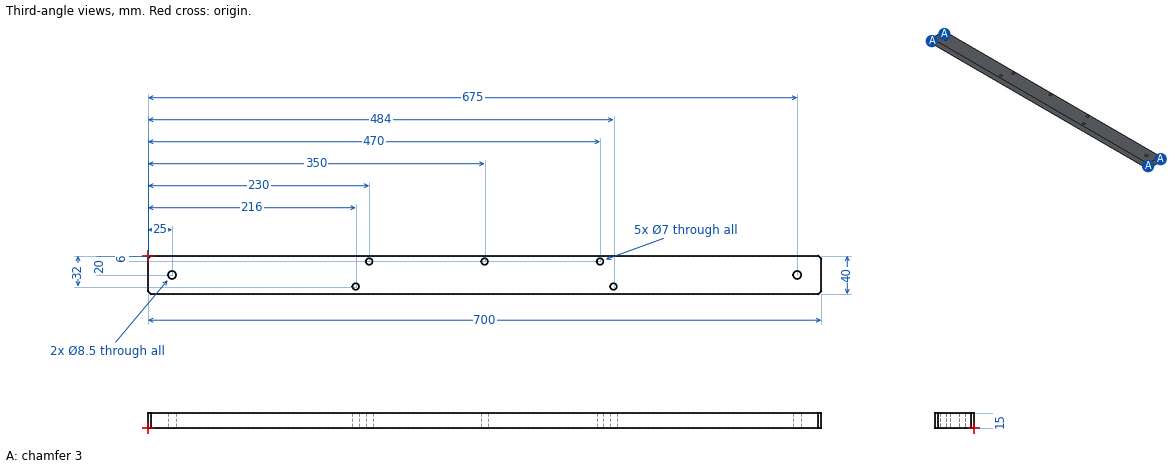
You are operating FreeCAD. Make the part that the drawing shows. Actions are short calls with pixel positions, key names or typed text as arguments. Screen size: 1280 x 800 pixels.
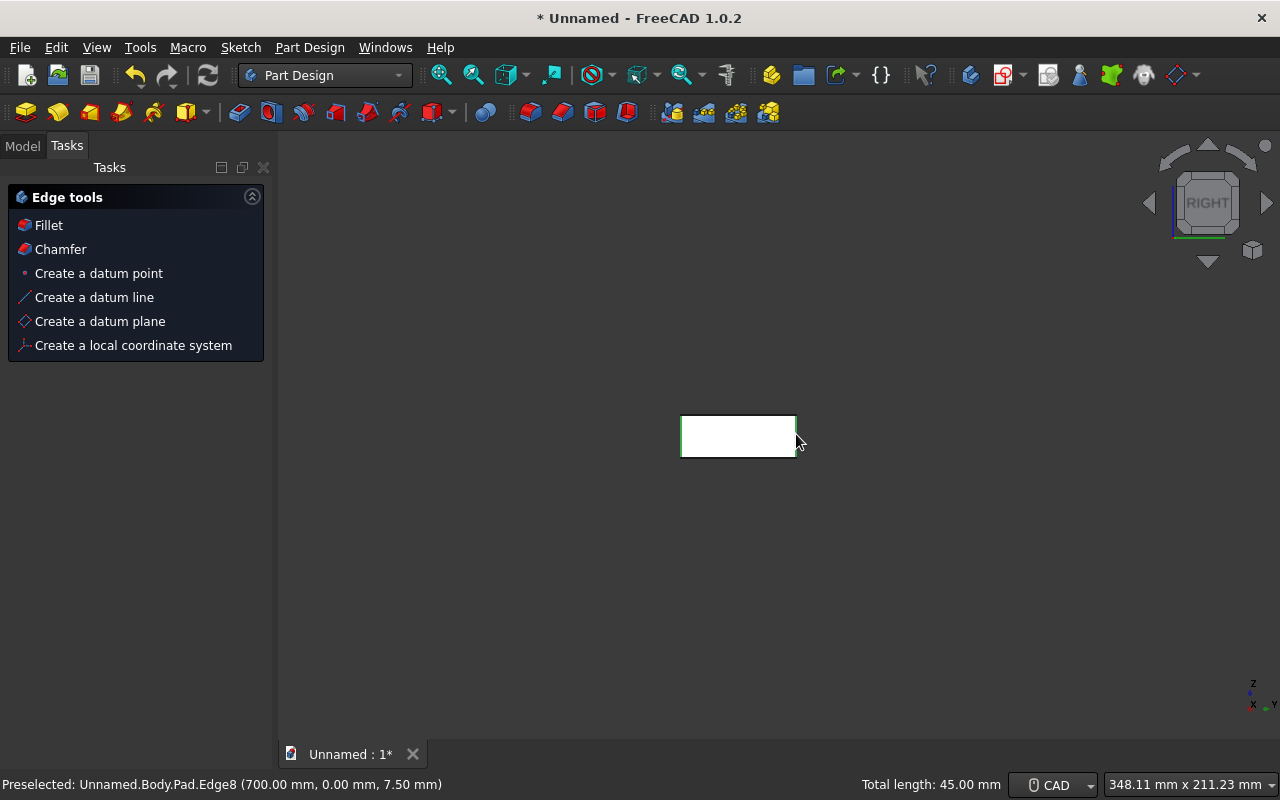
click(442, 76)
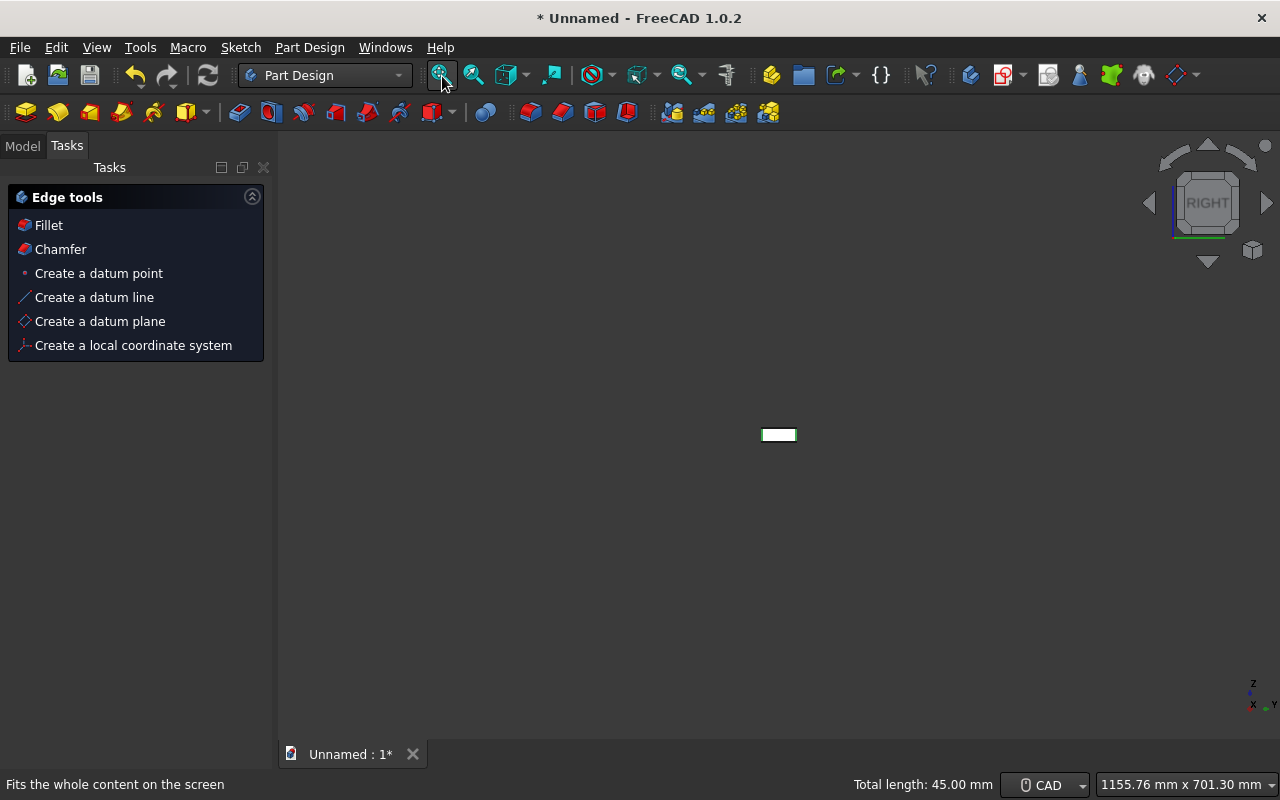
key(5)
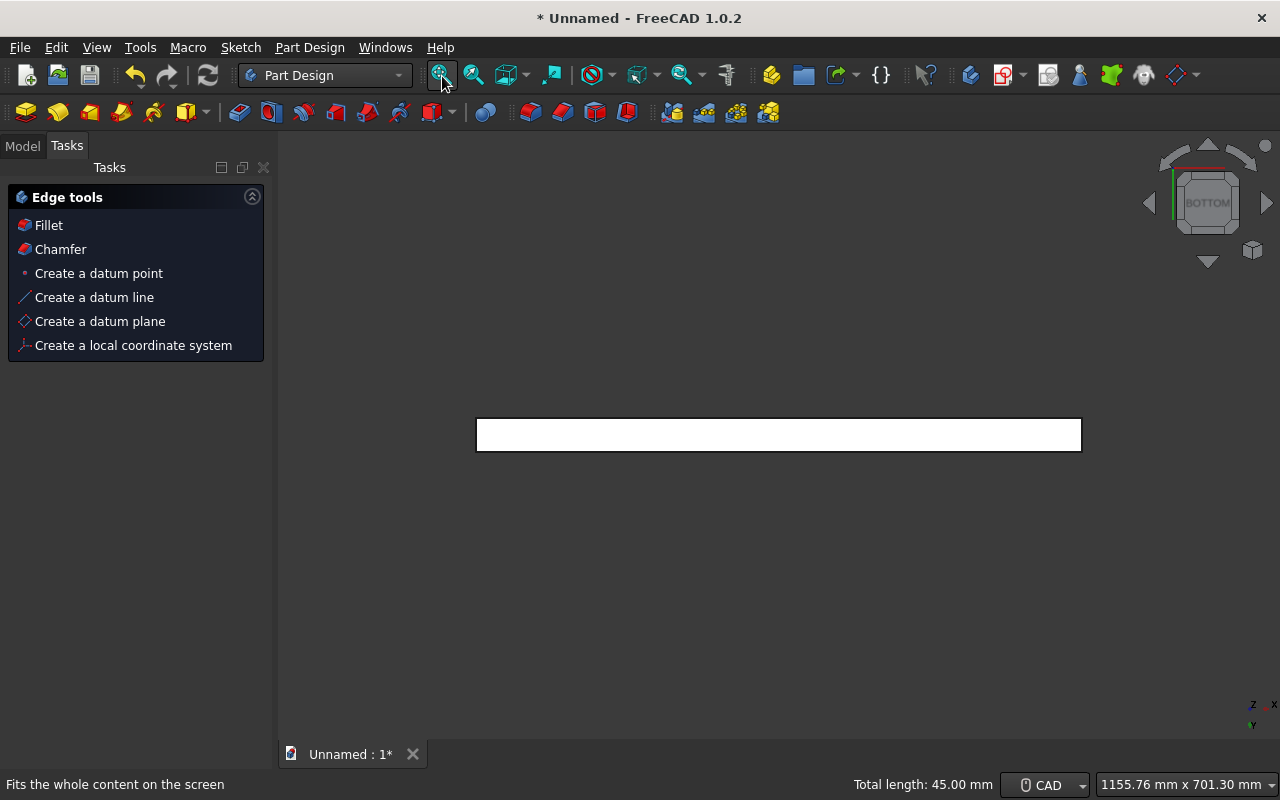
scroll(476, 451, up, 6)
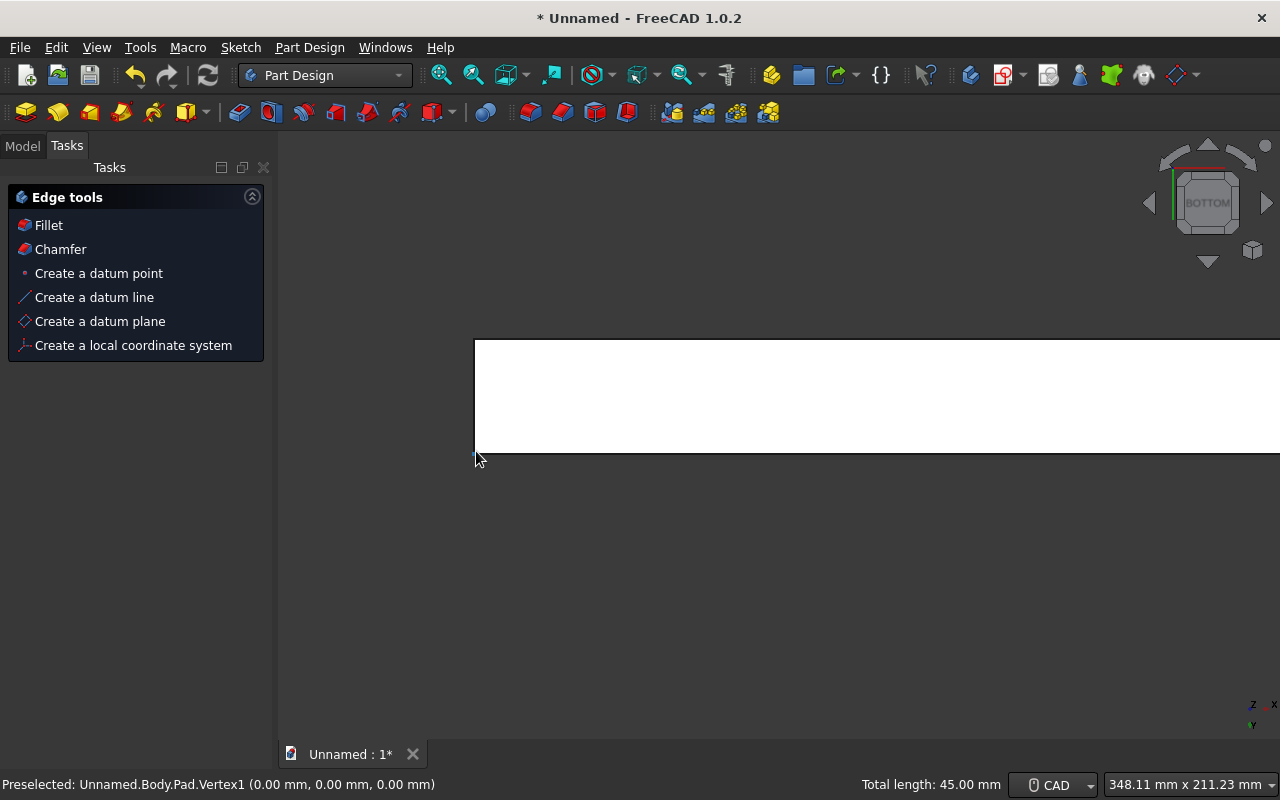
click(442, 76)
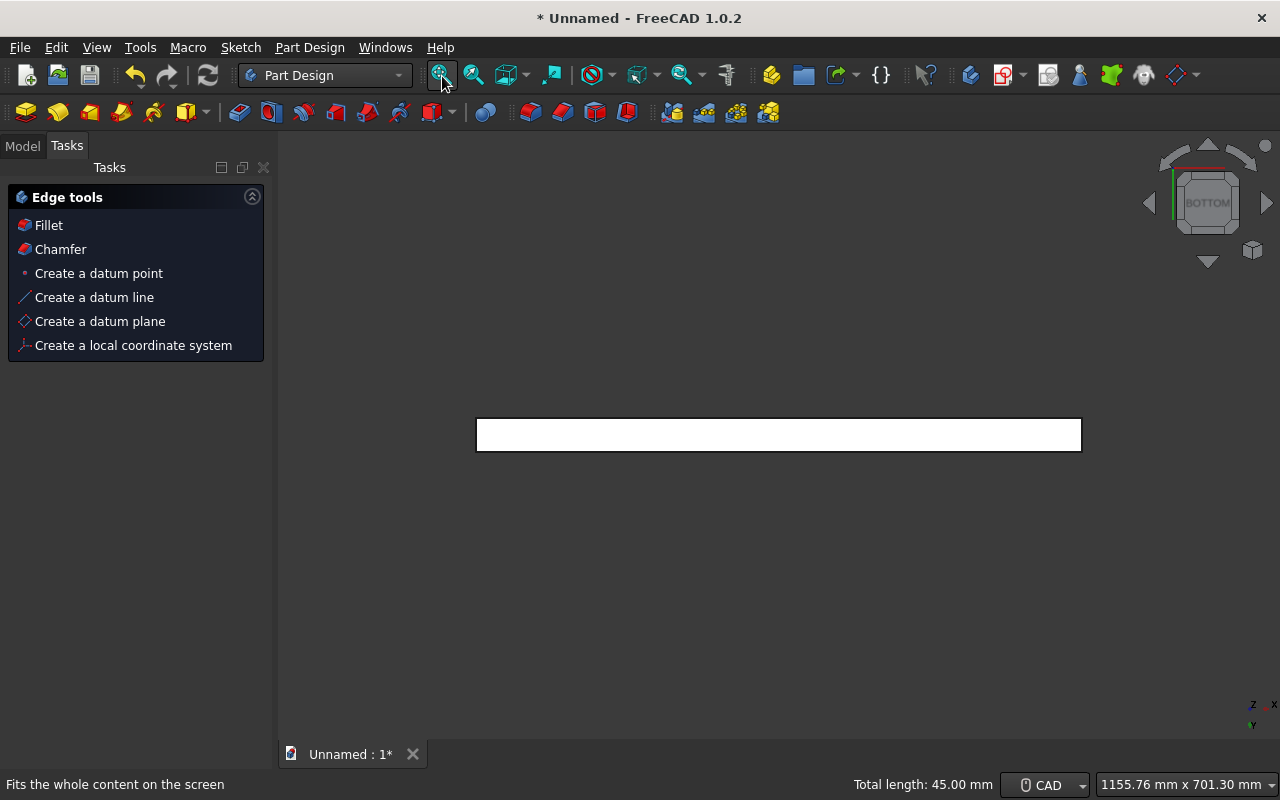
key(4)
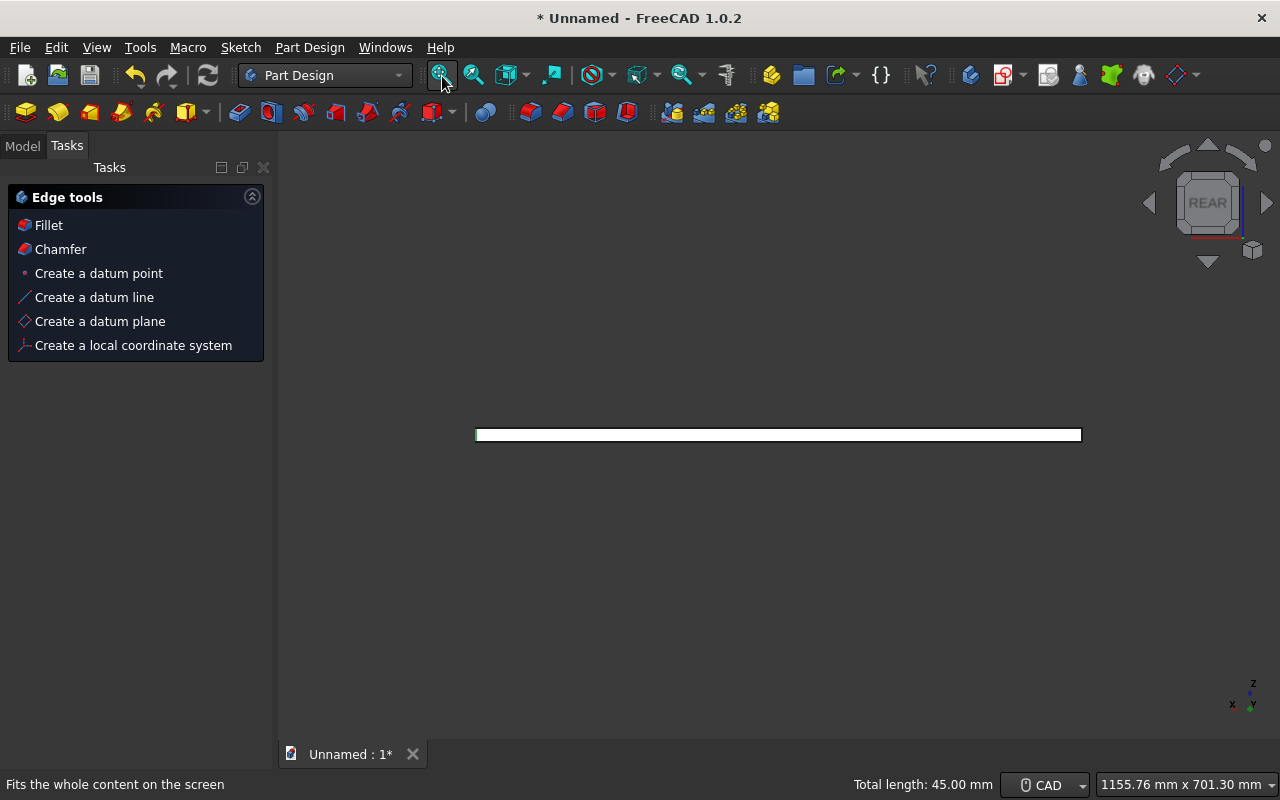
click(1082, 434, ctrl)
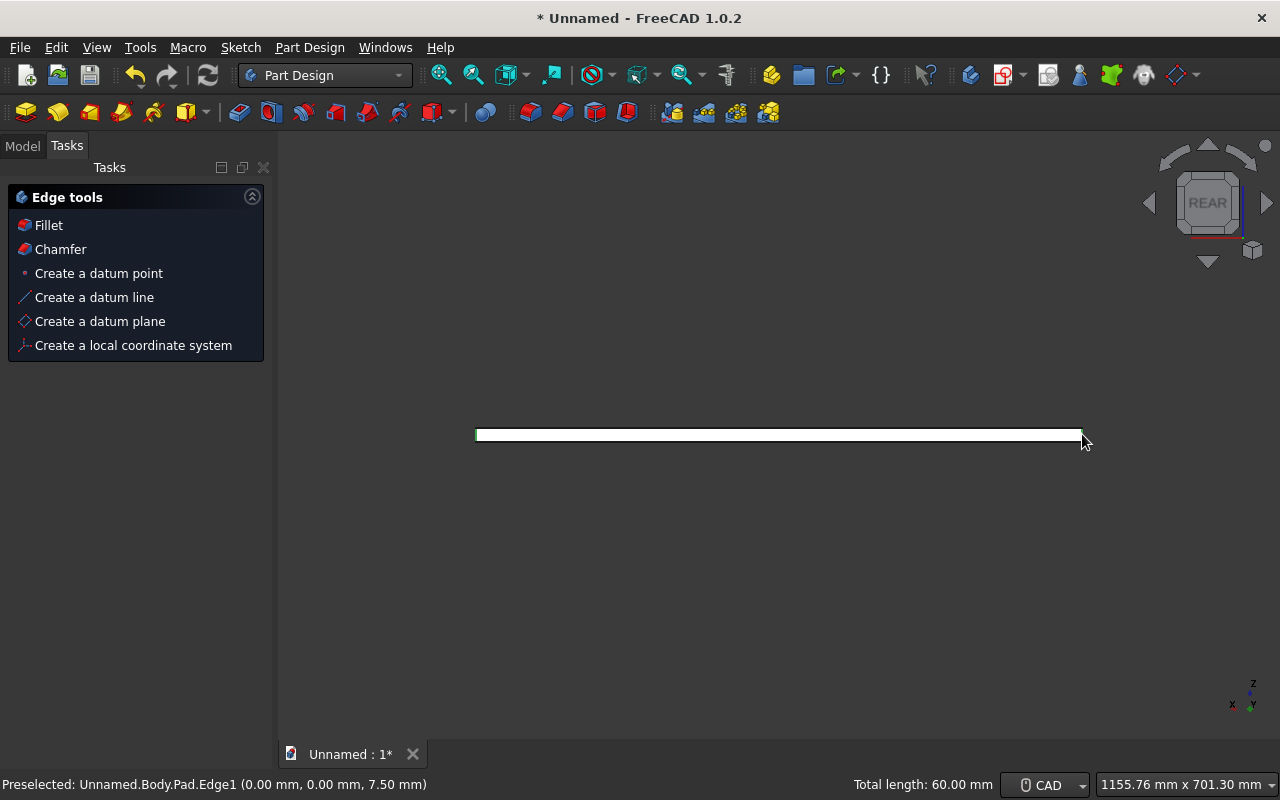
click(564, 112)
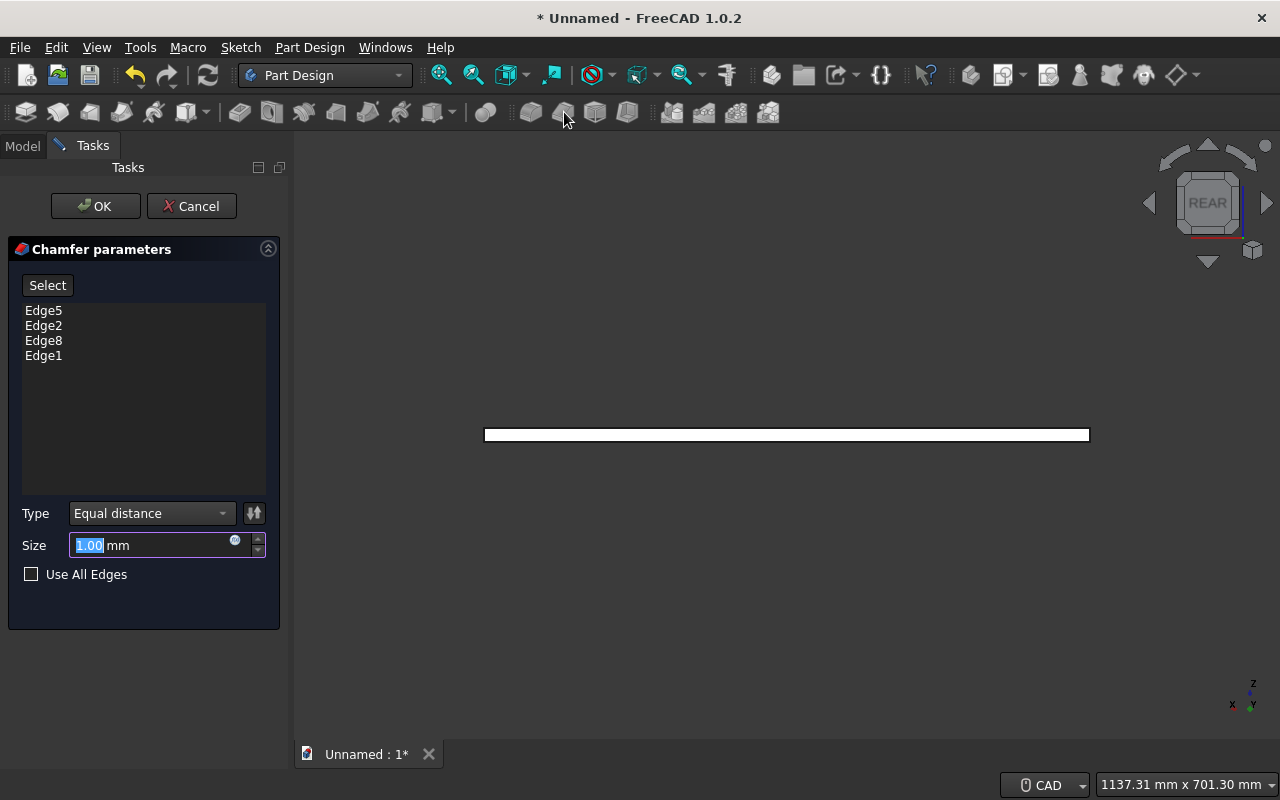
text(3)
key(Tab)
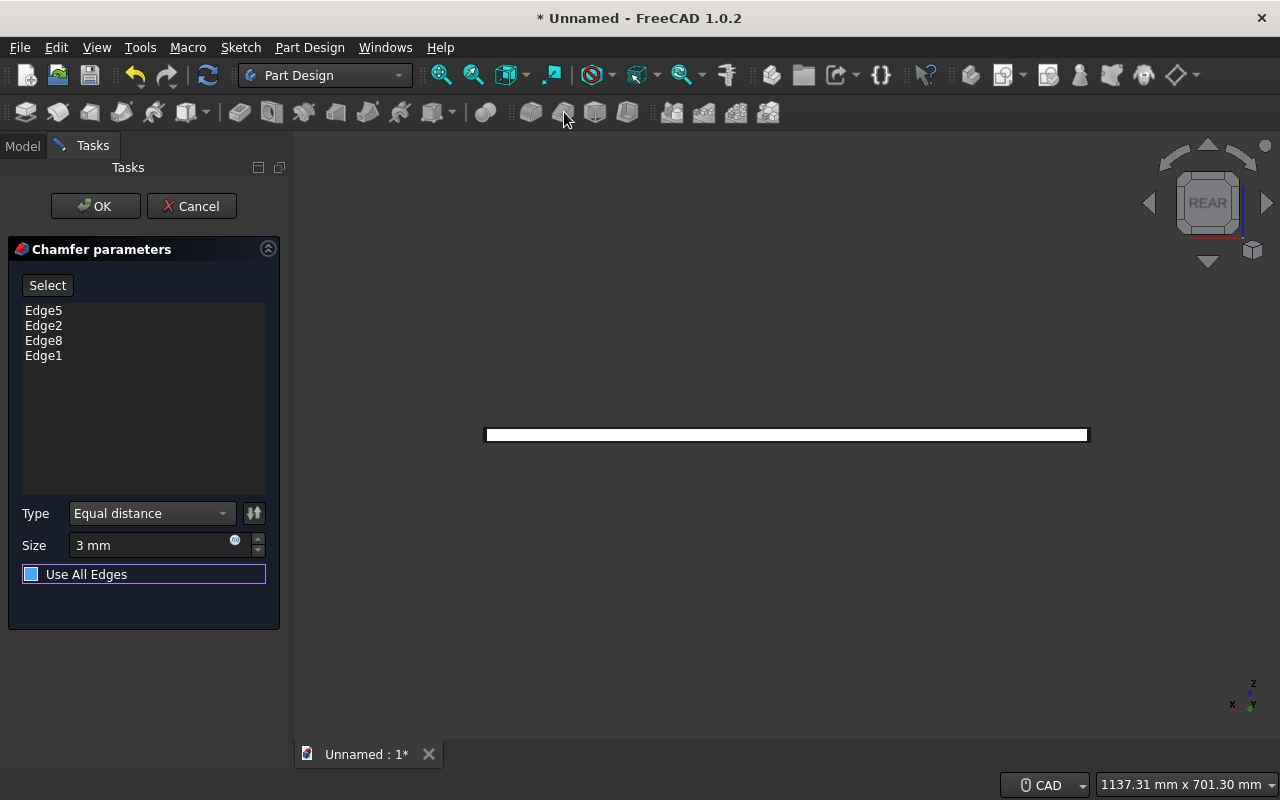
click(96, 206)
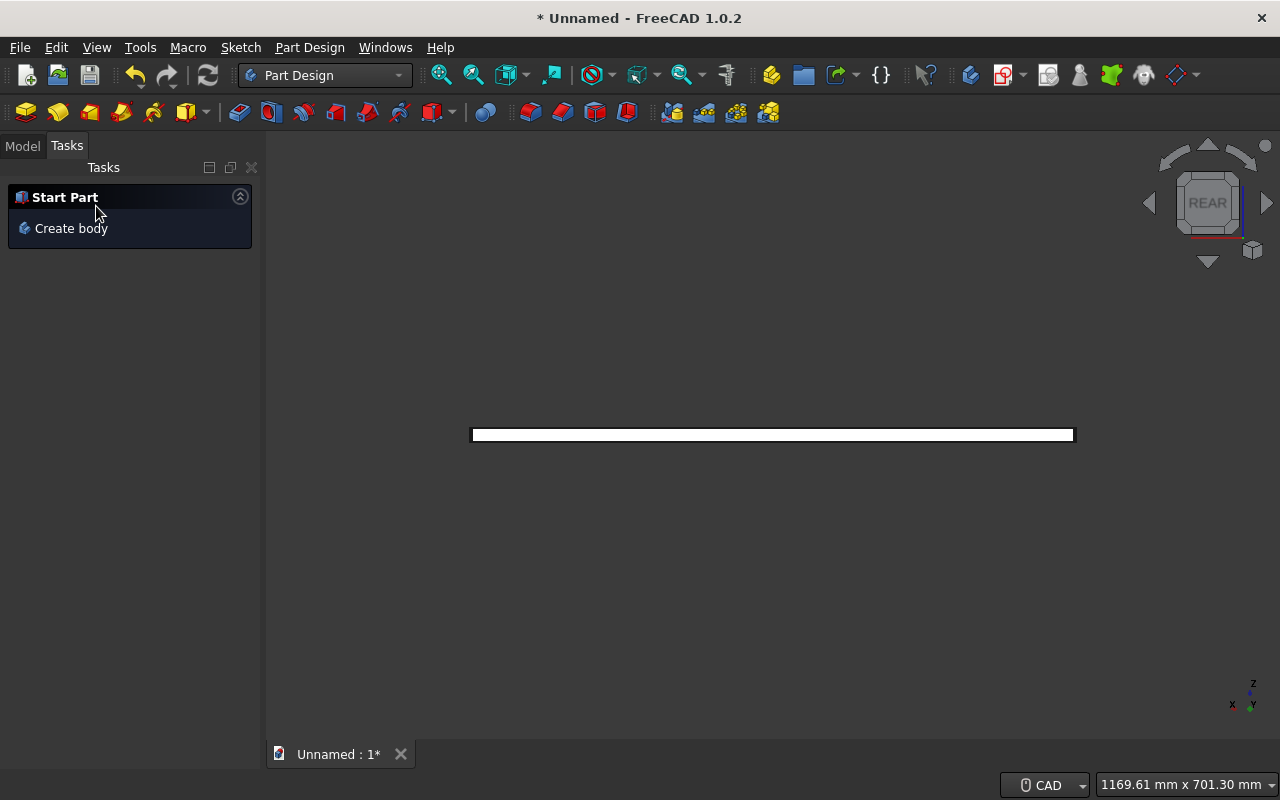
key(0)